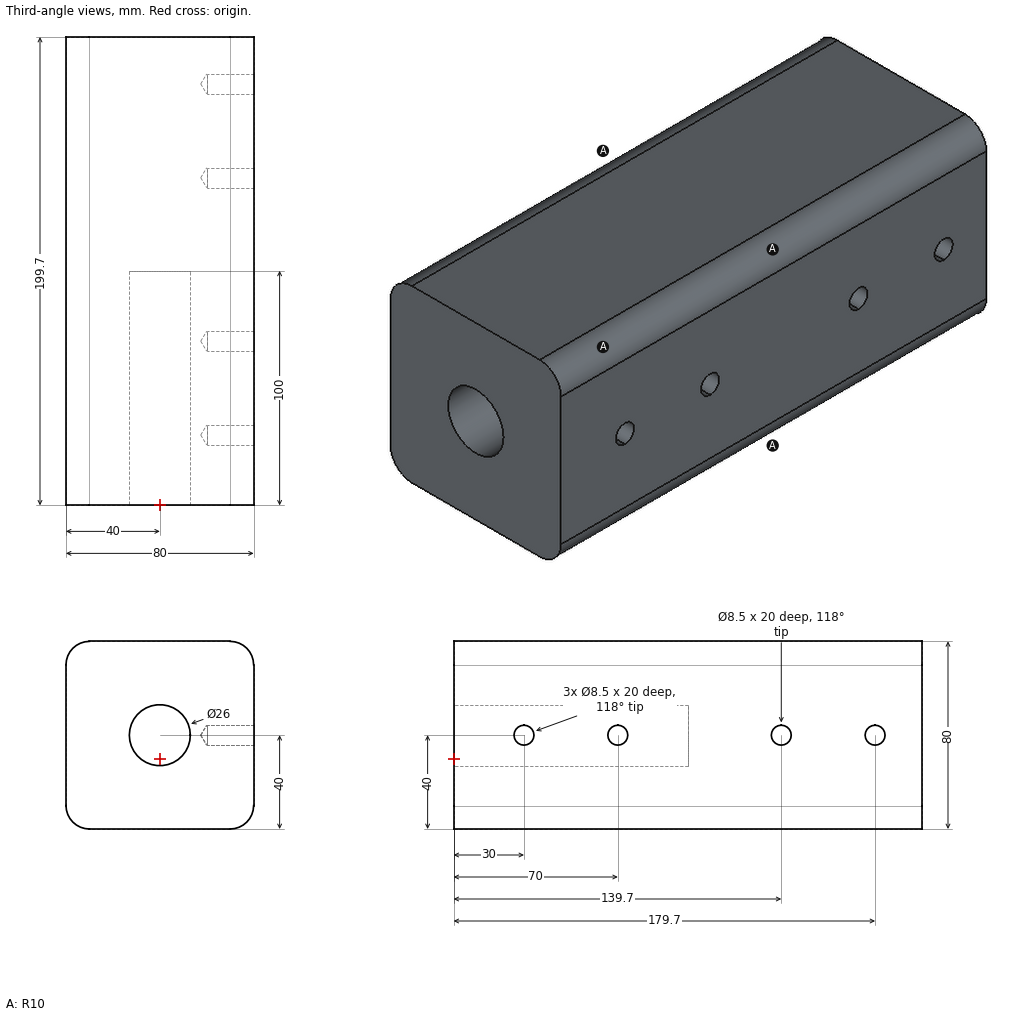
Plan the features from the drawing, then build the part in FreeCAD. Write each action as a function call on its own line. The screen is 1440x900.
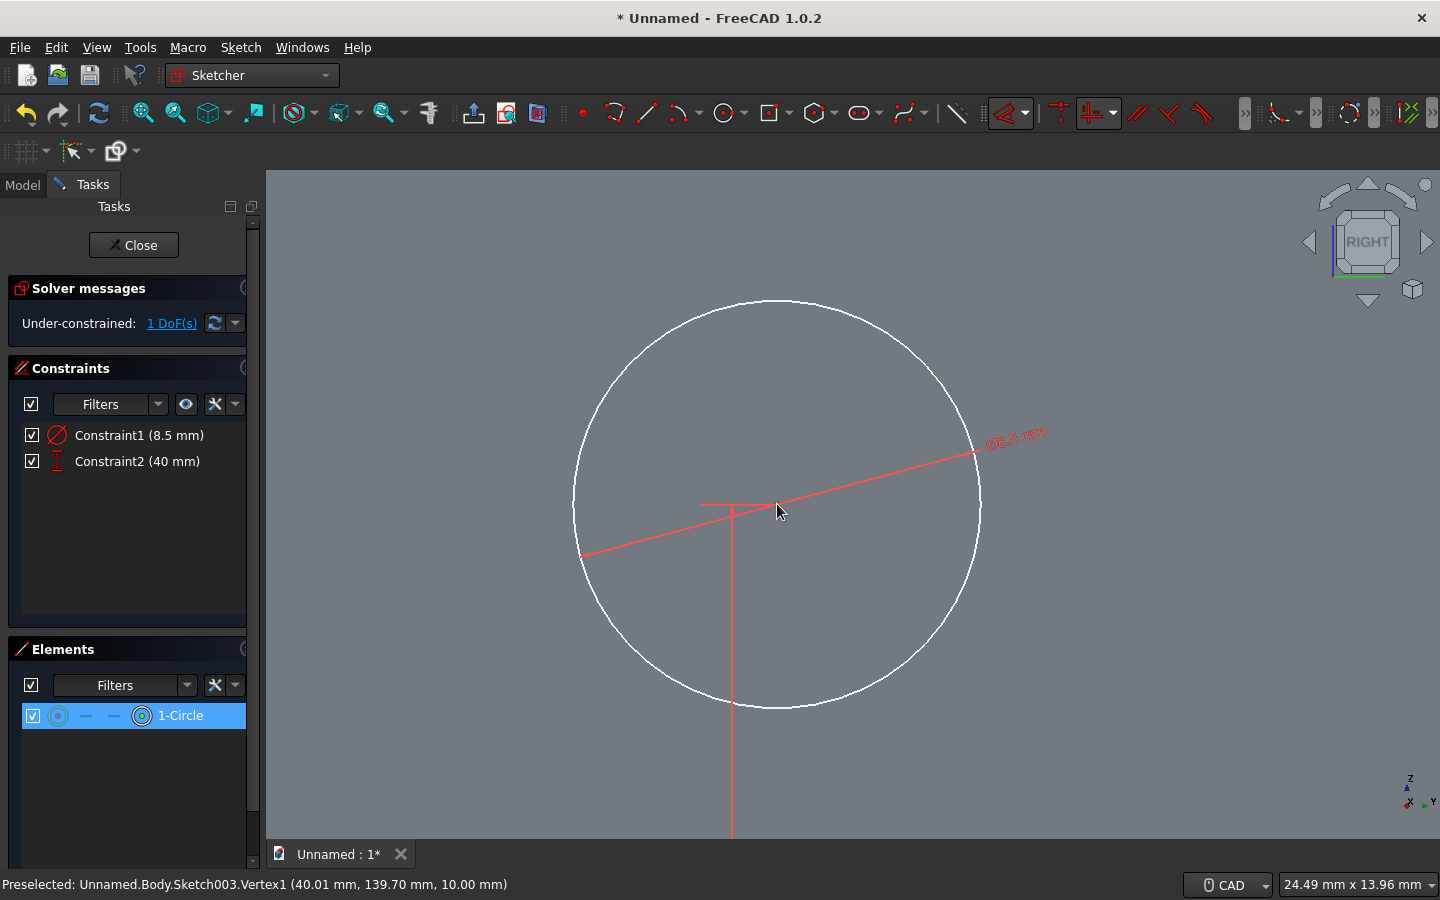
key(l)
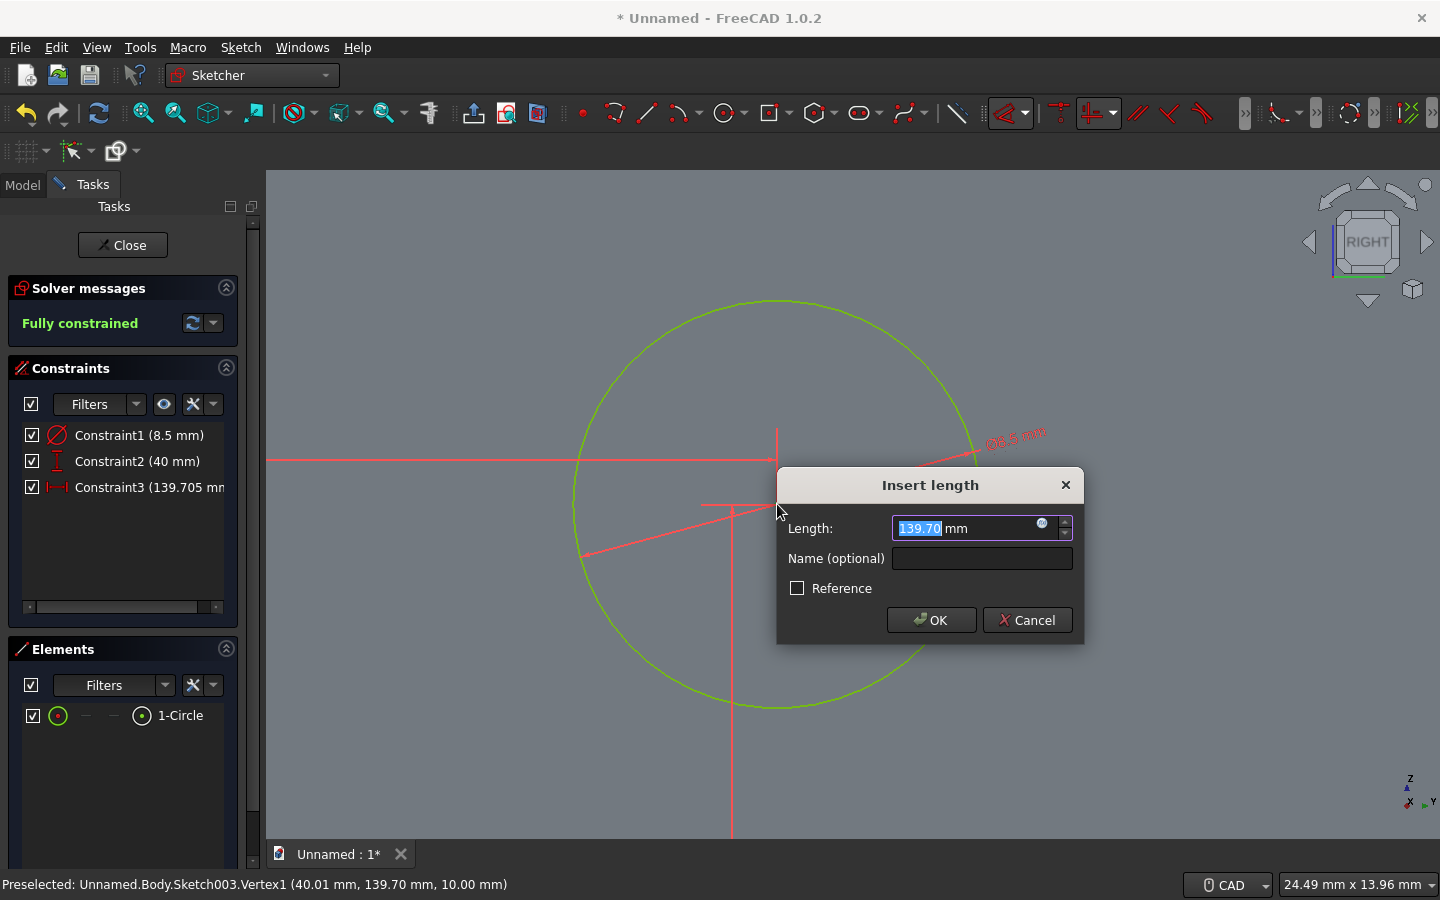
text(139.7)
key(Return)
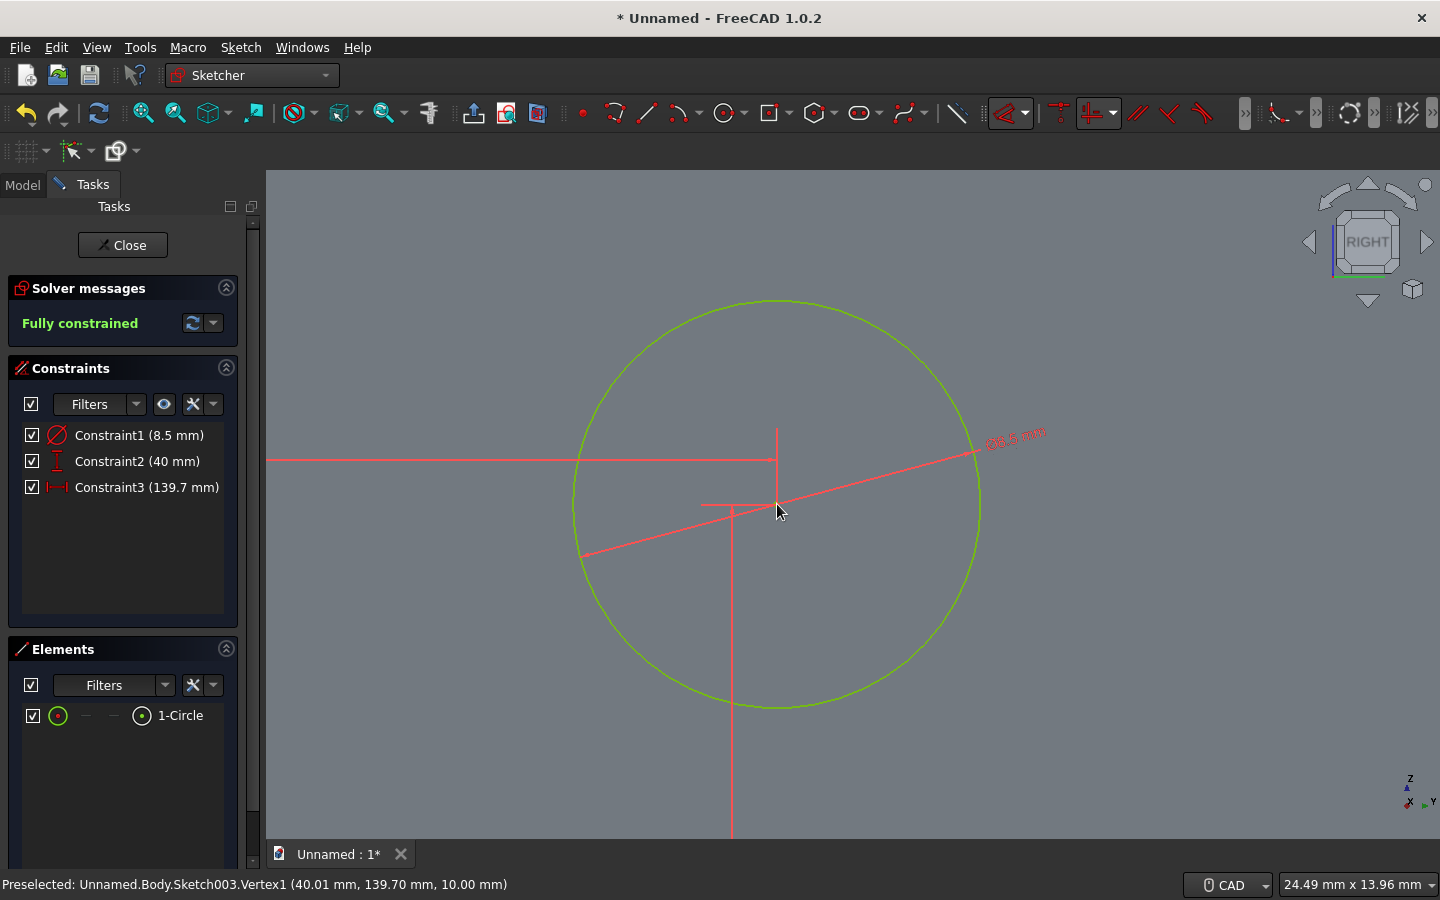
click(123, 245)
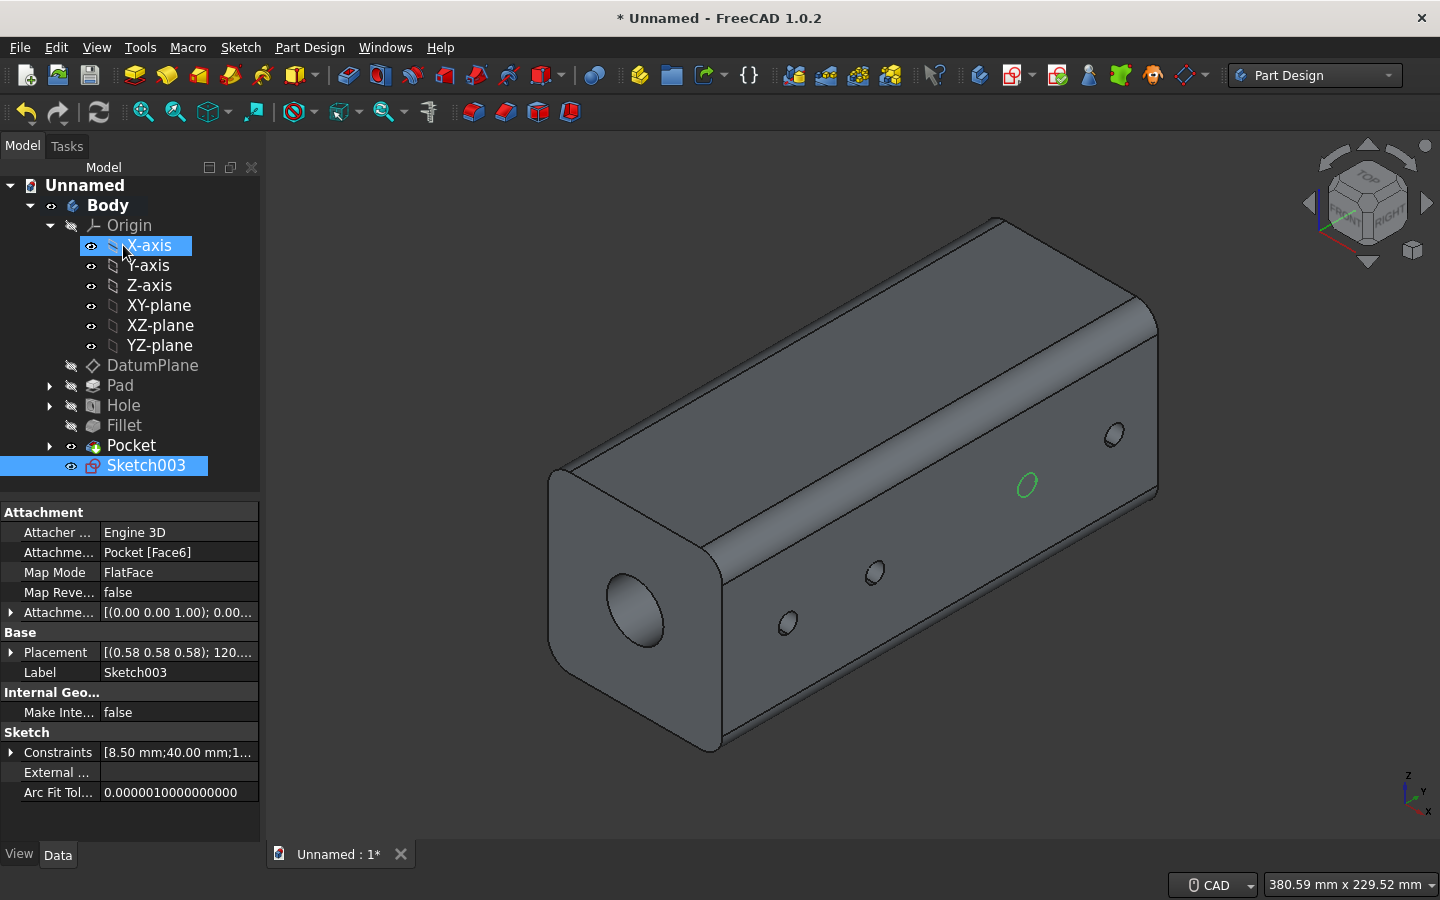
click(382, 76)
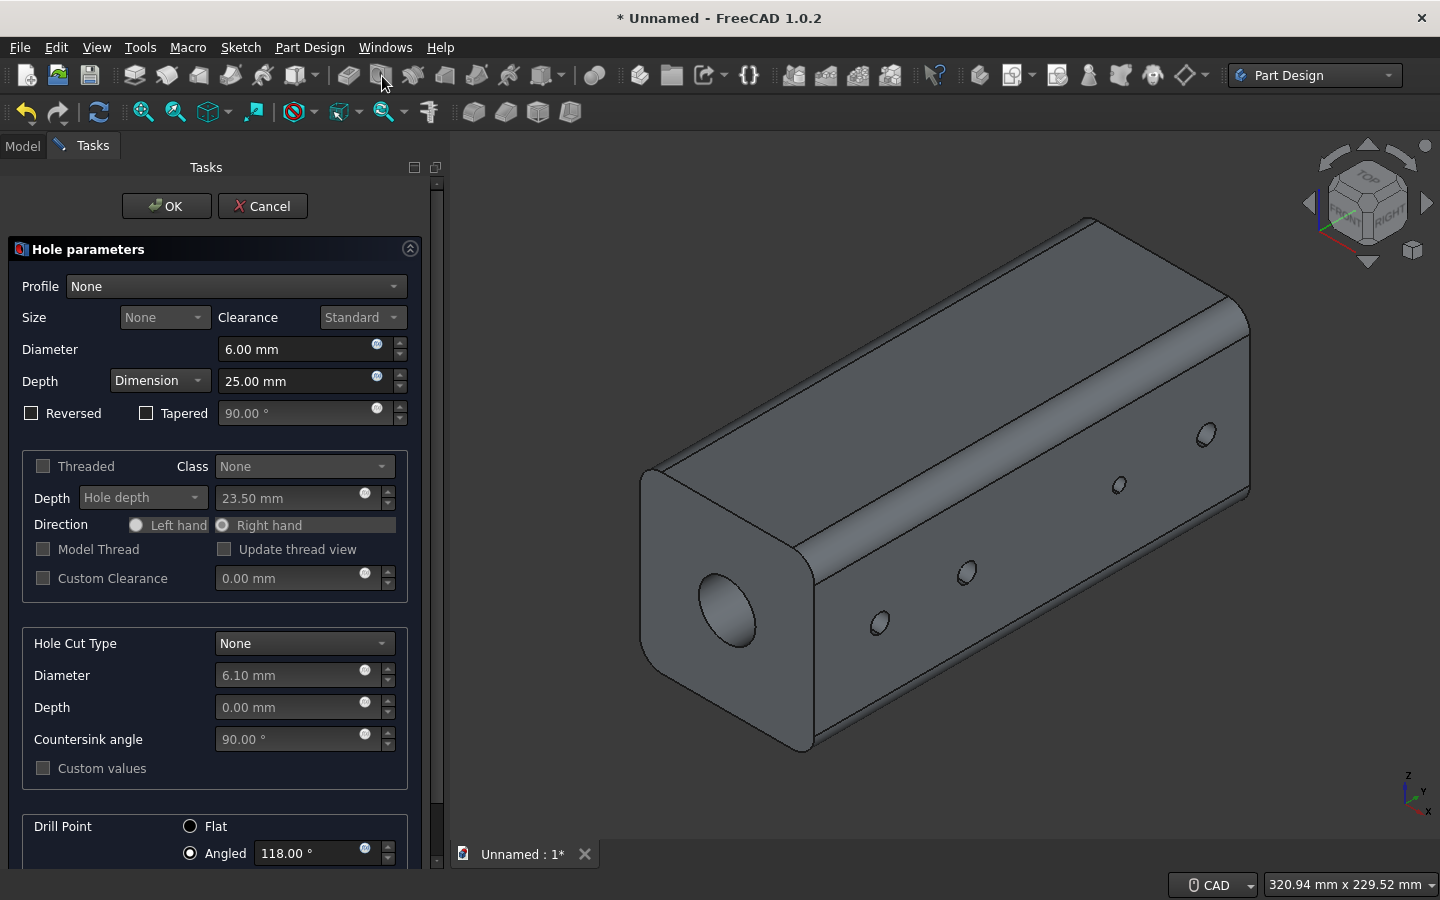
triple_click(305, 349)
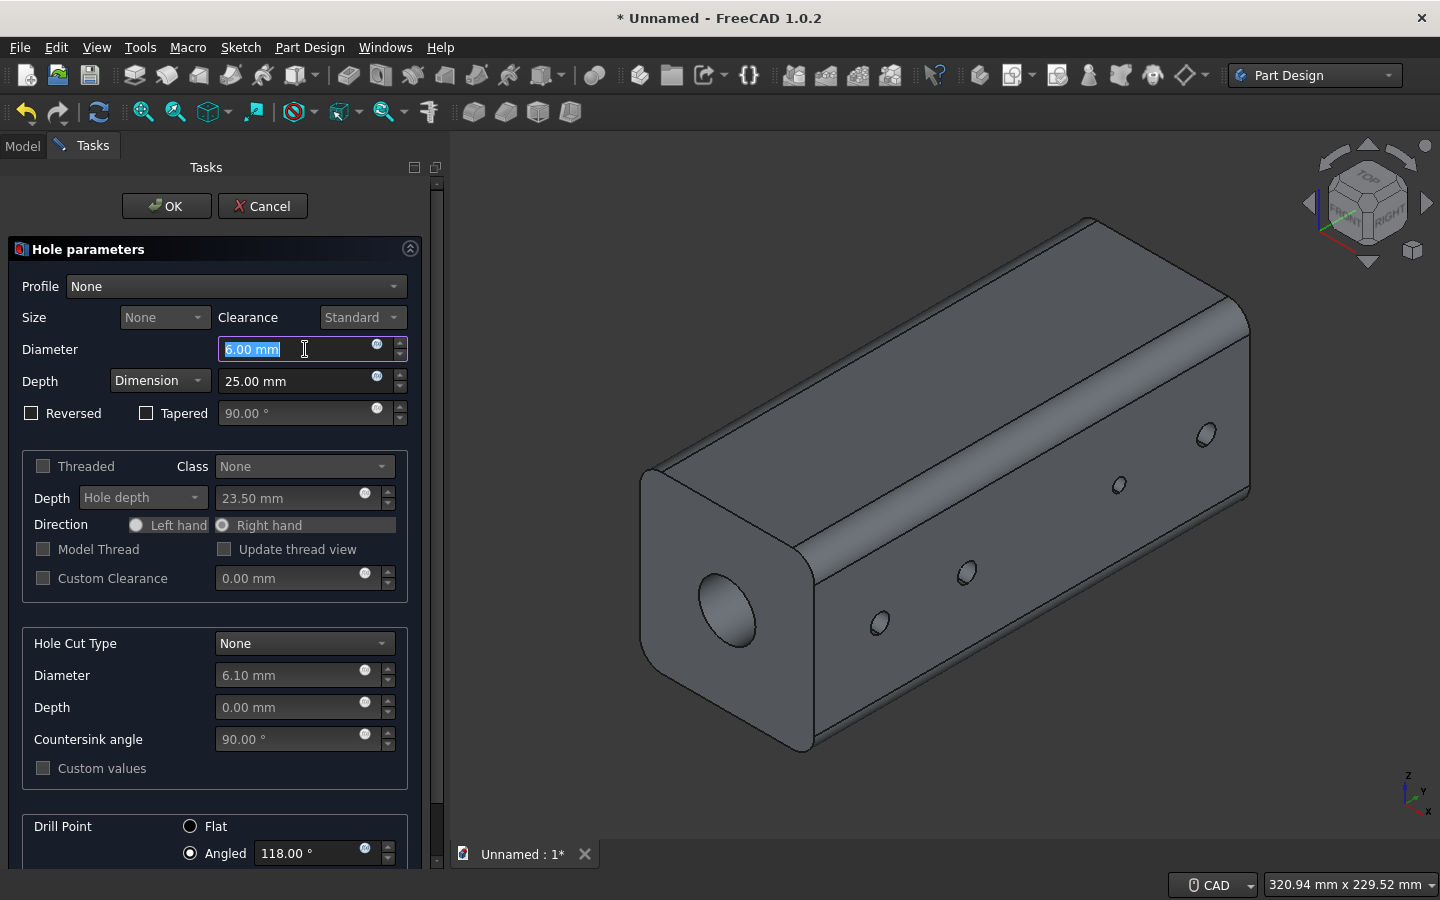
text(8.5)
key(Tab)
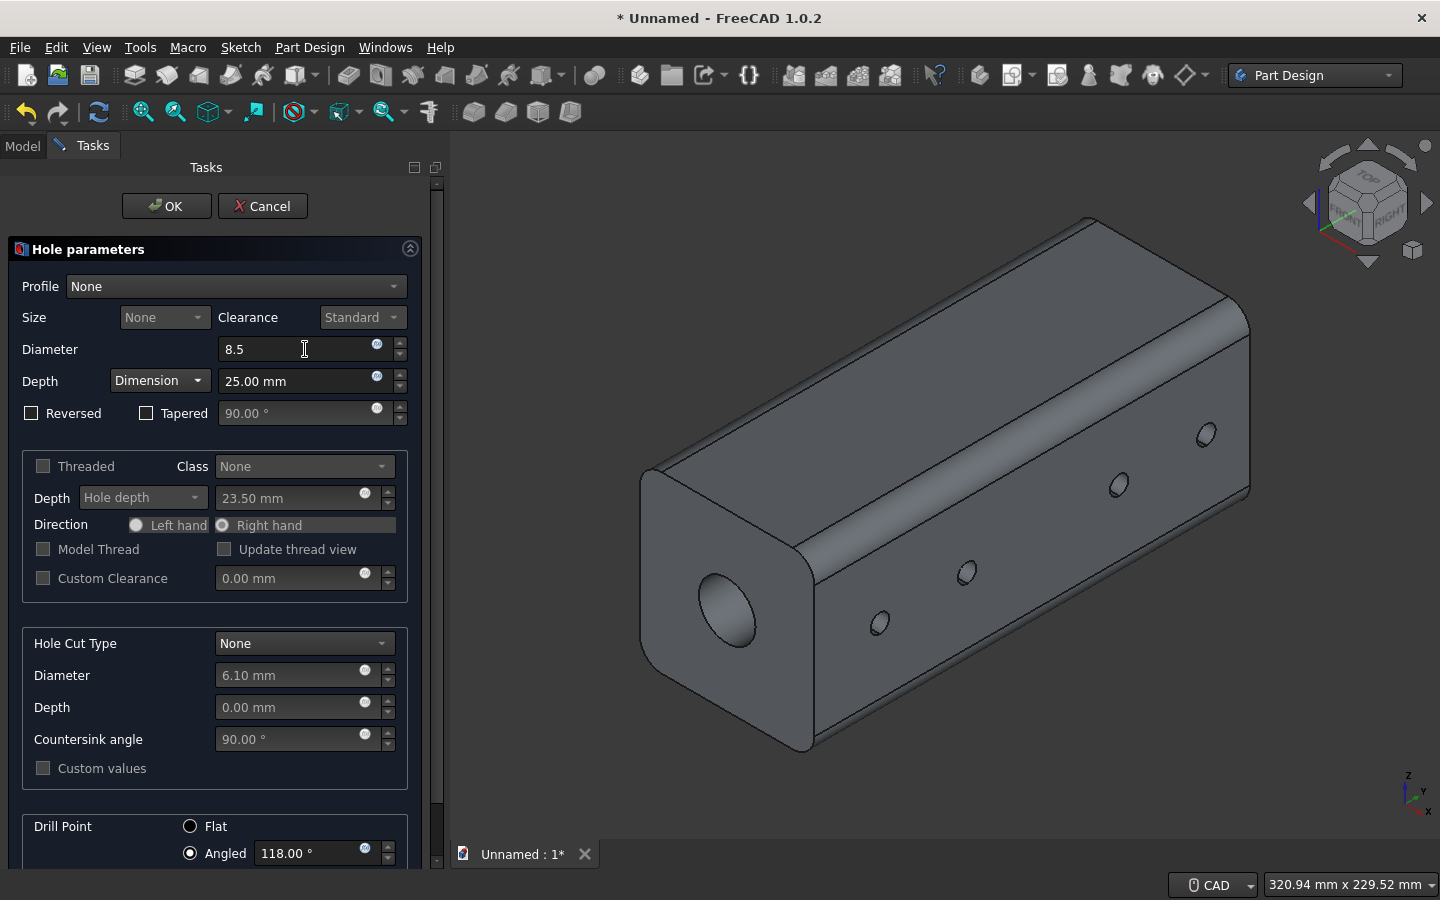
triple_click(305, 381)